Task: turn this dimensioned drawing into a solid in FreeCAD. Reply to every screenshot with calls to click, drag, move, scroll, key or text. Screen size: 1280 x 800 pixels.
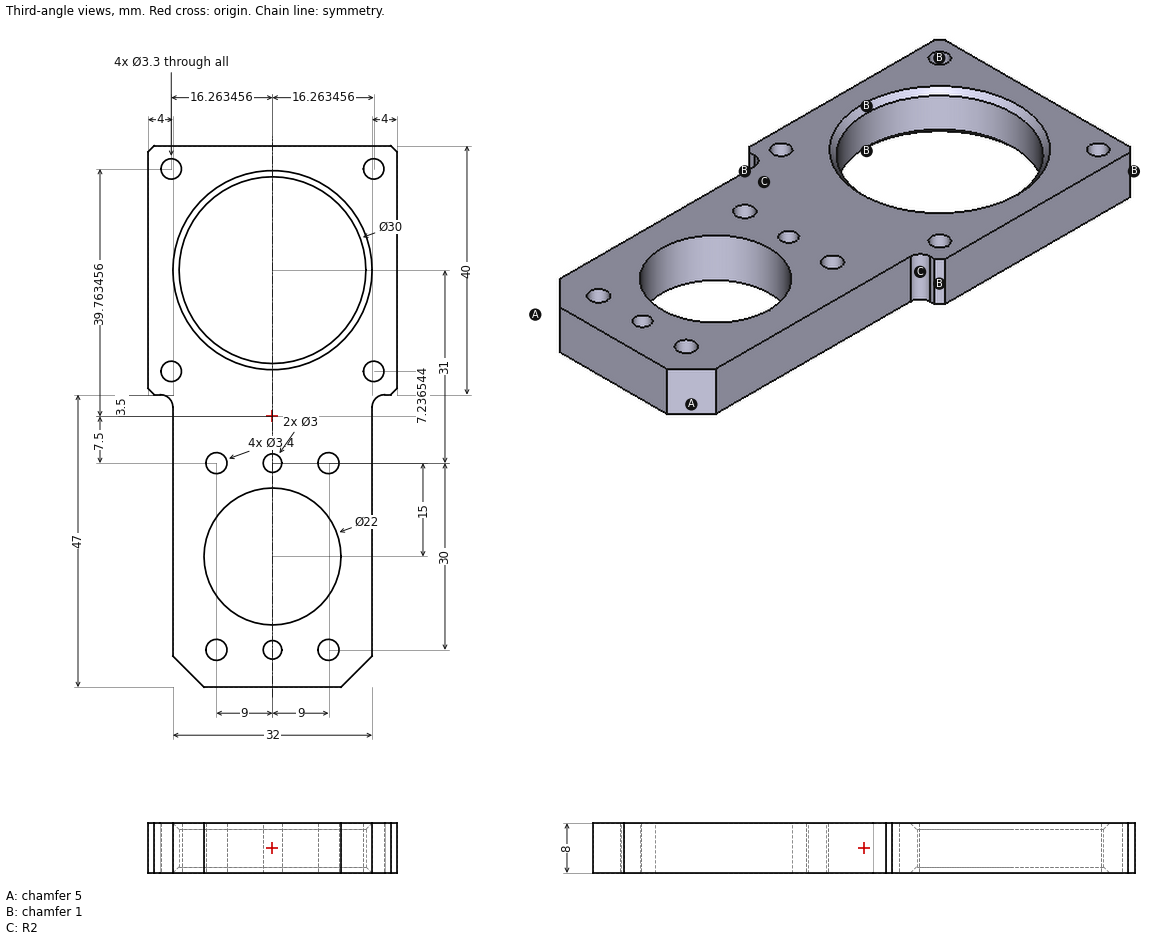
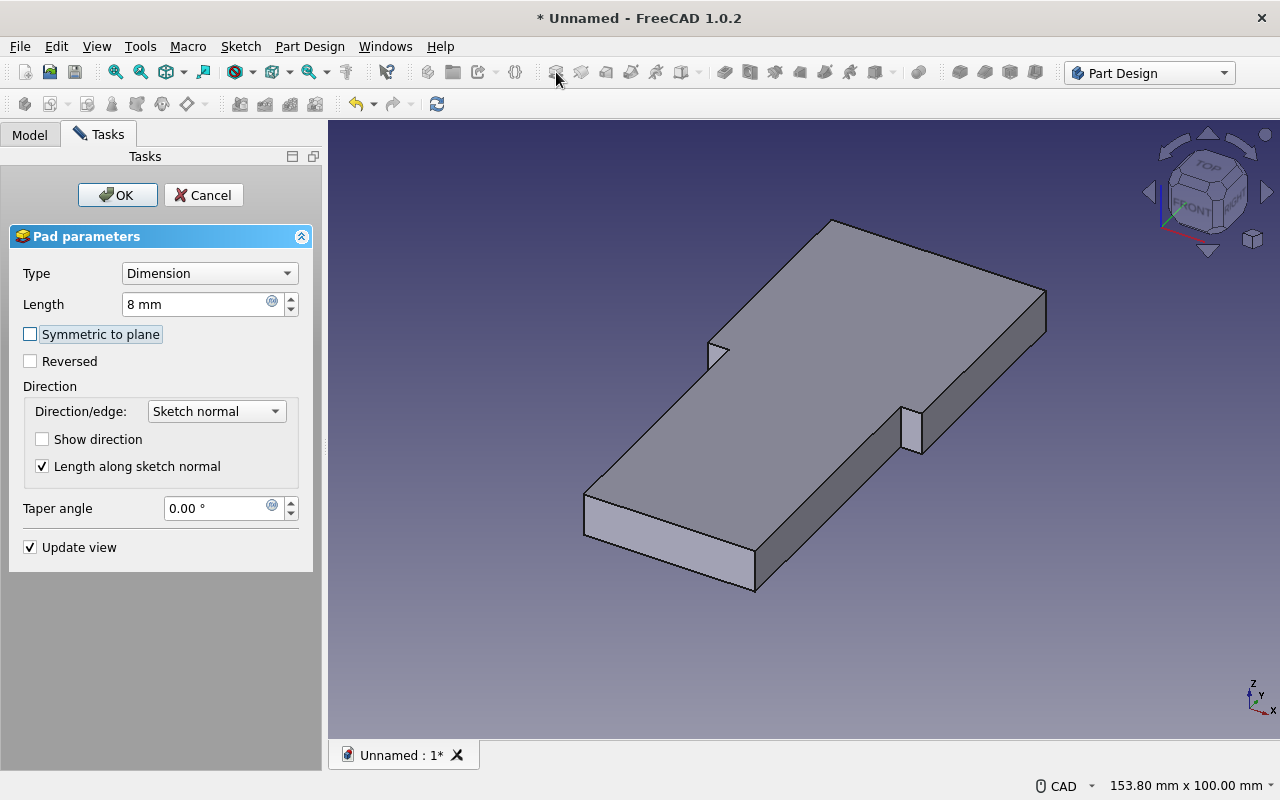
click(31, 334)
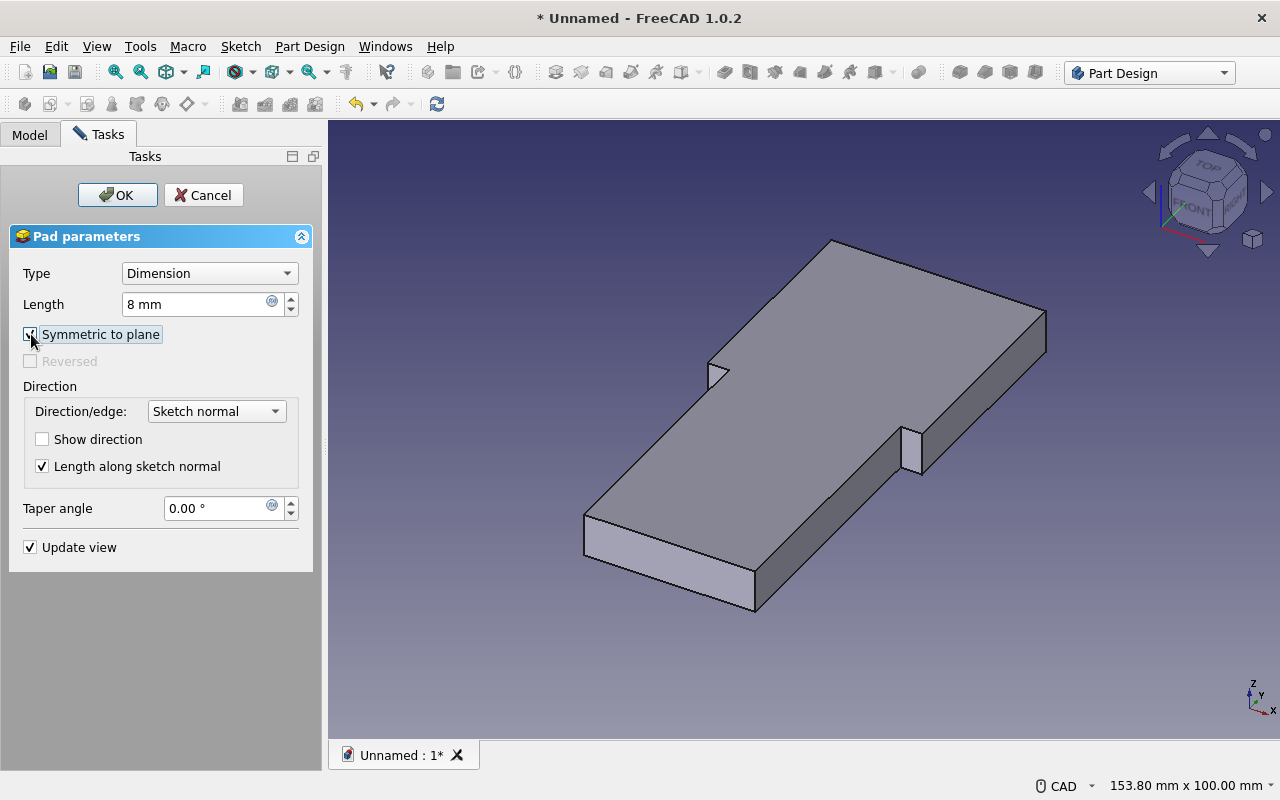
click(118, 195)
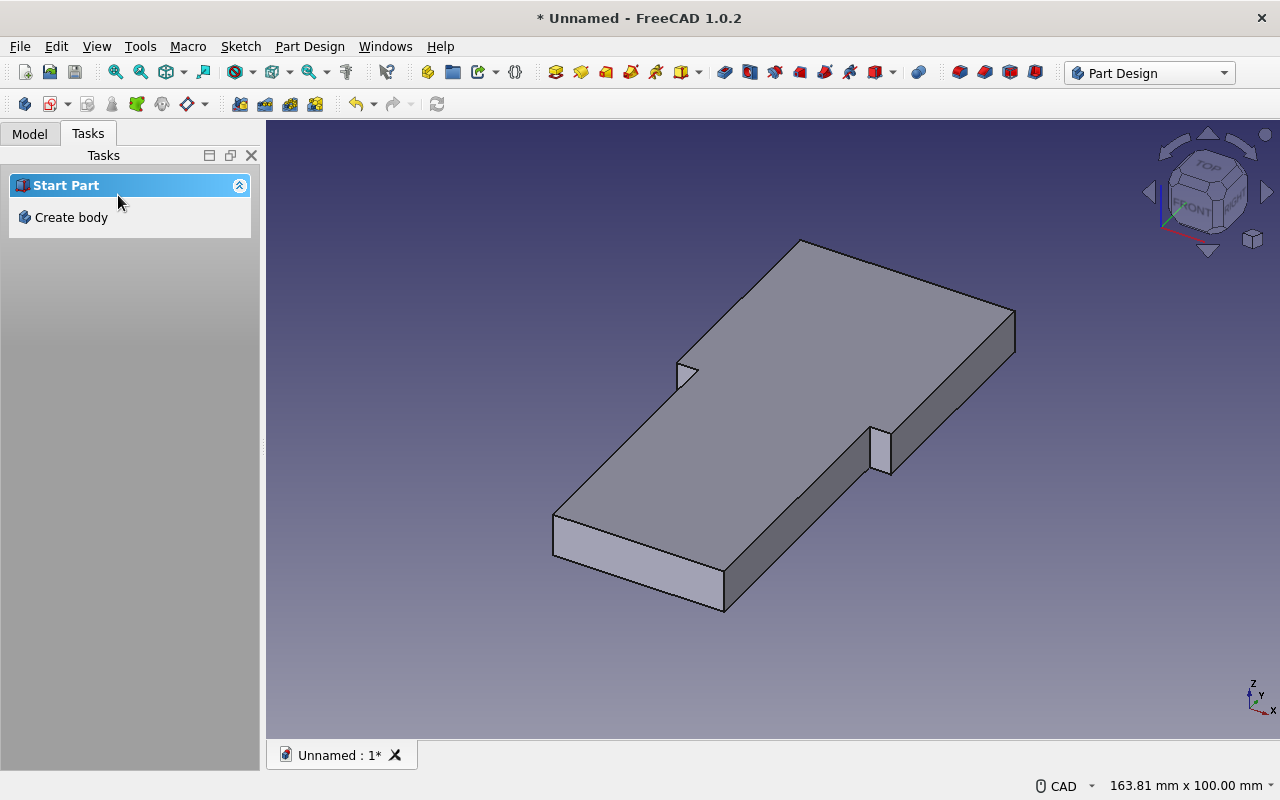
click(850, 332)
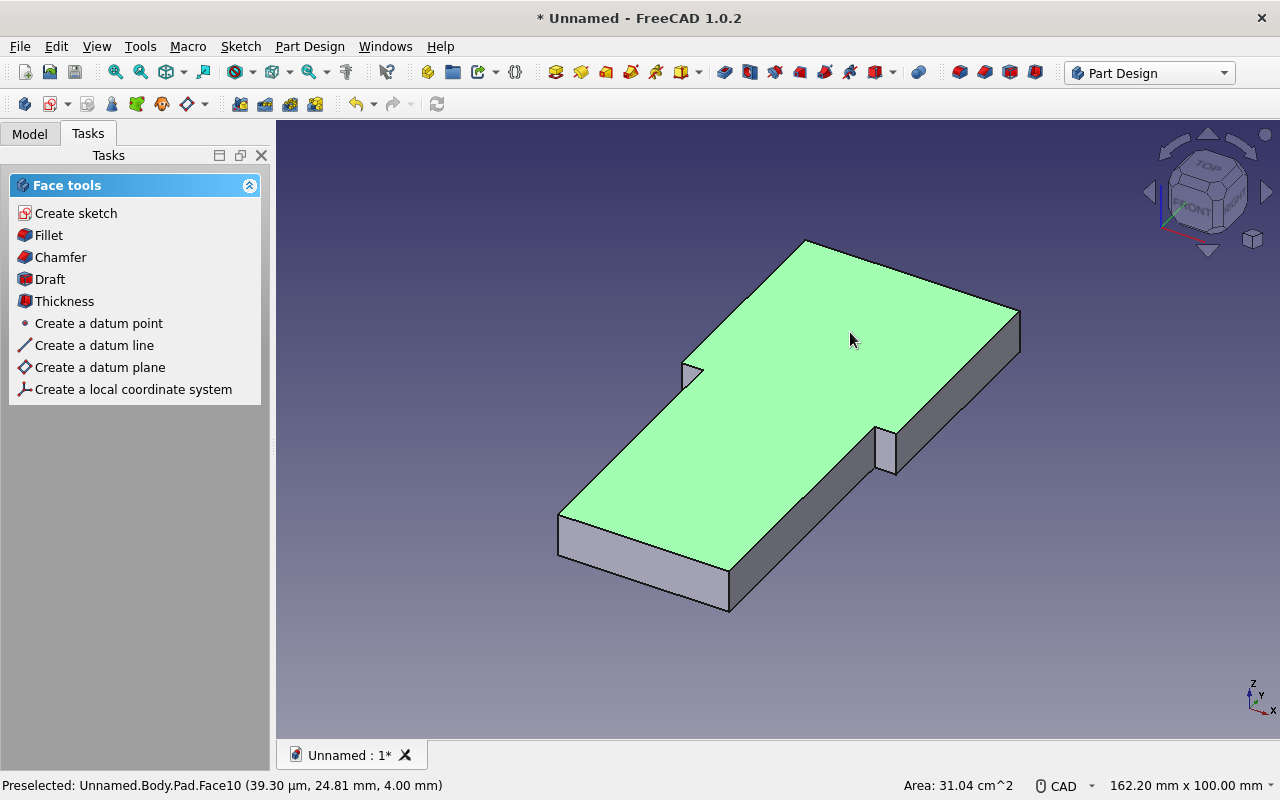
click(50, 104)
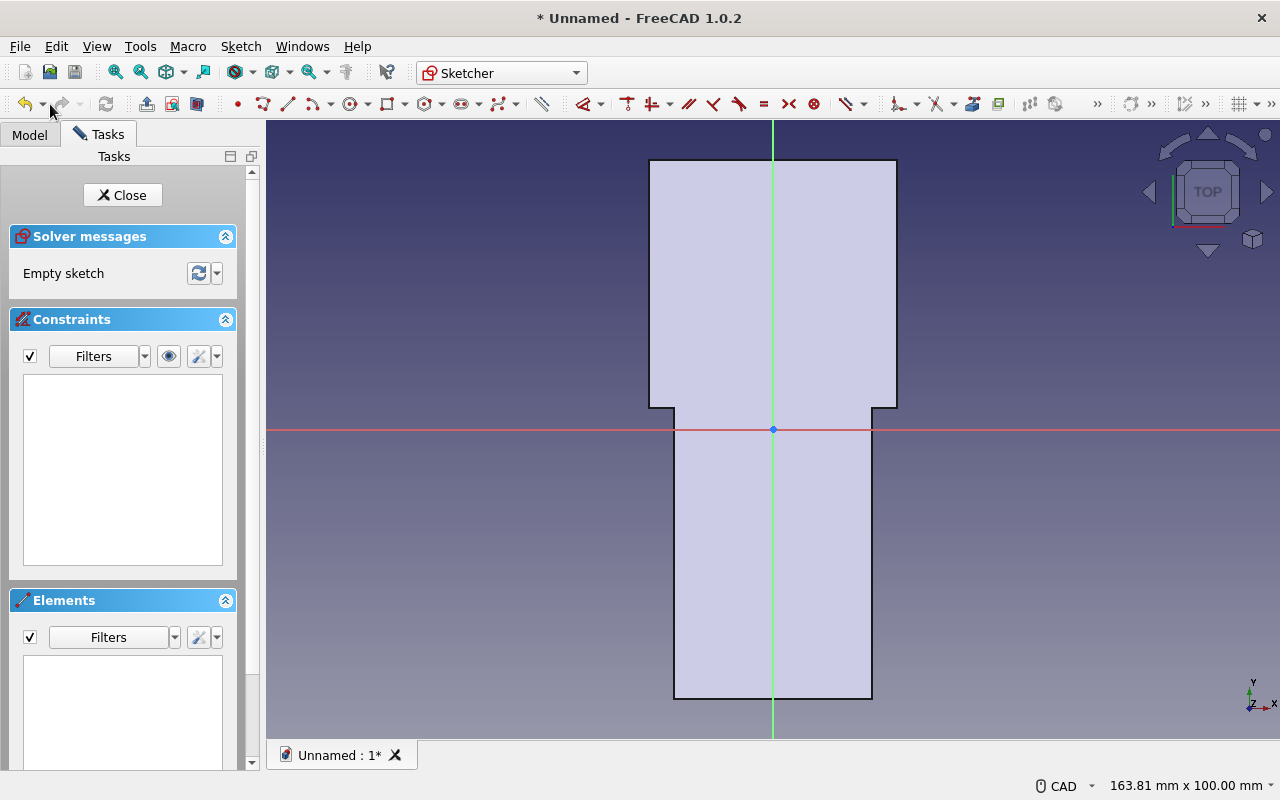
scroll(912, 148, up, 2)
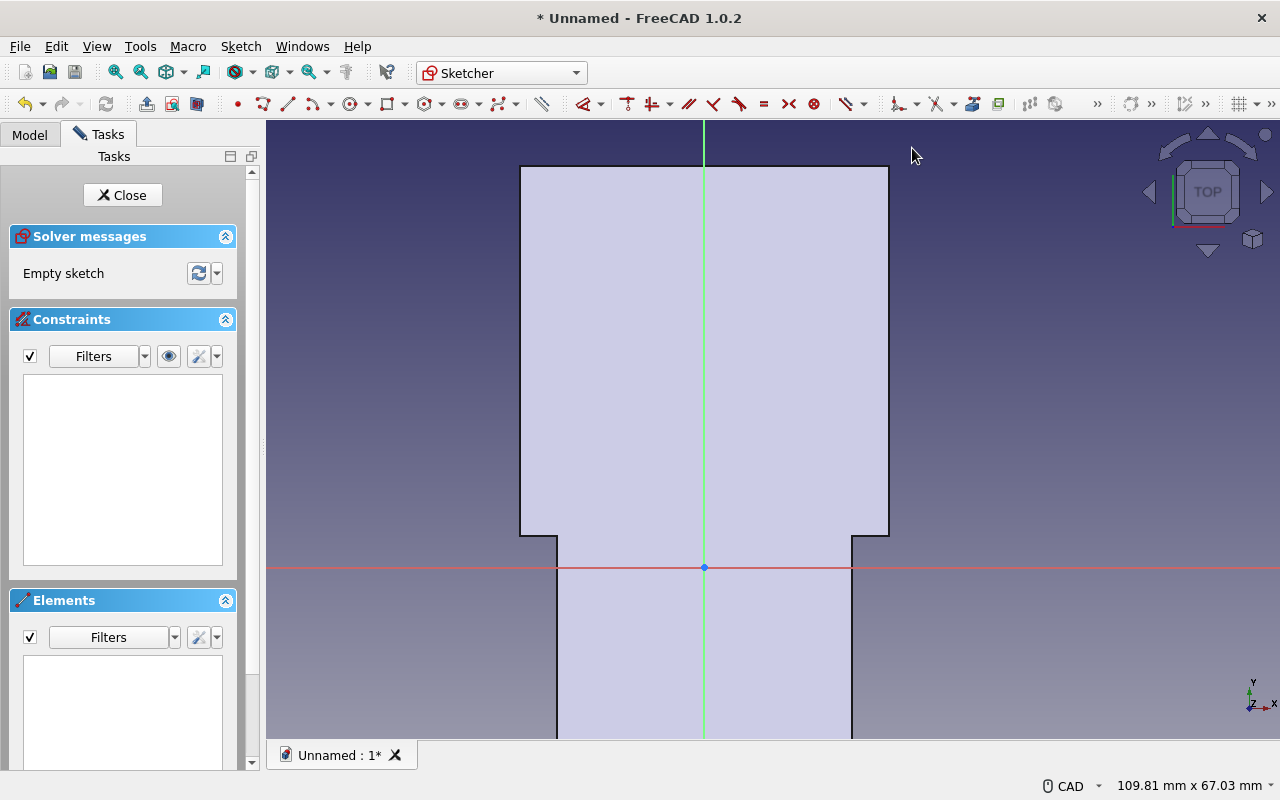
click(350, 104)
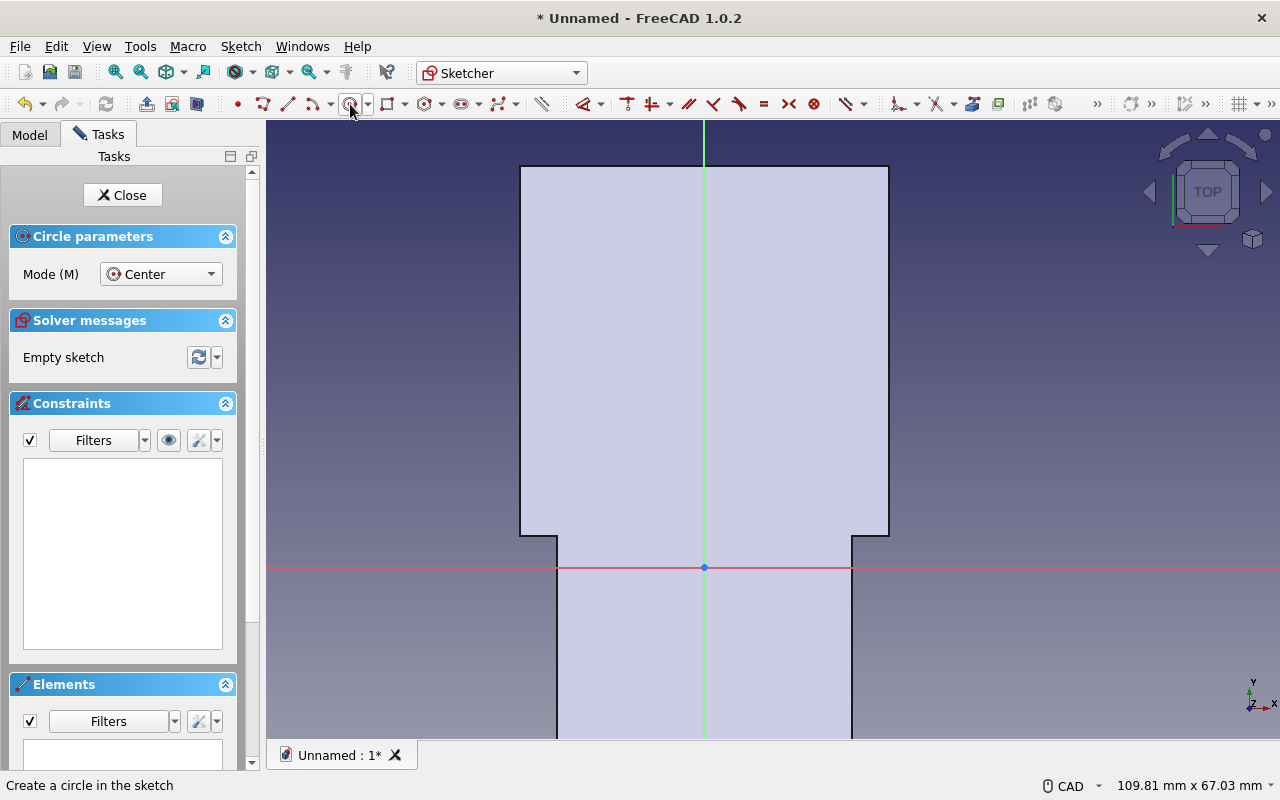
scroll(554, 201, up, 2)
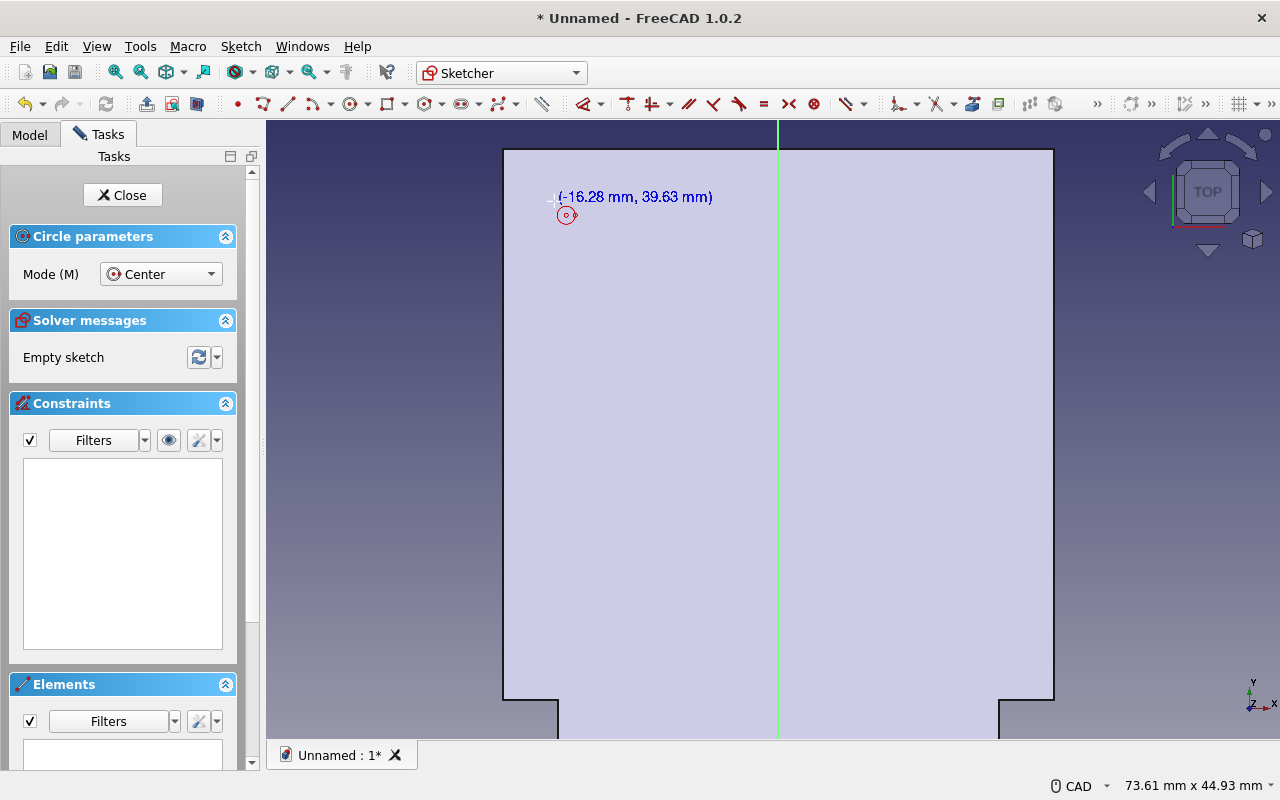
click(554, 201)
click(570, 184)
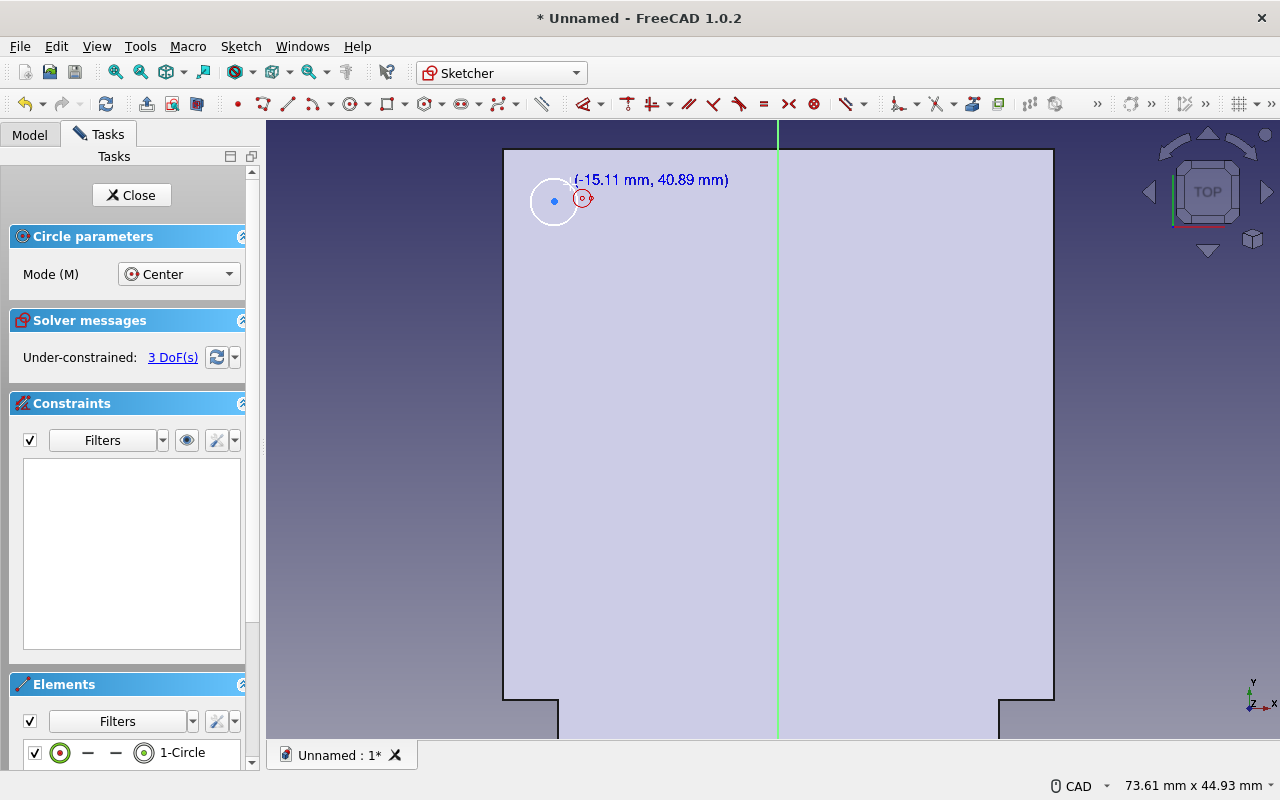
click(1002, 201)
click(1018, 184)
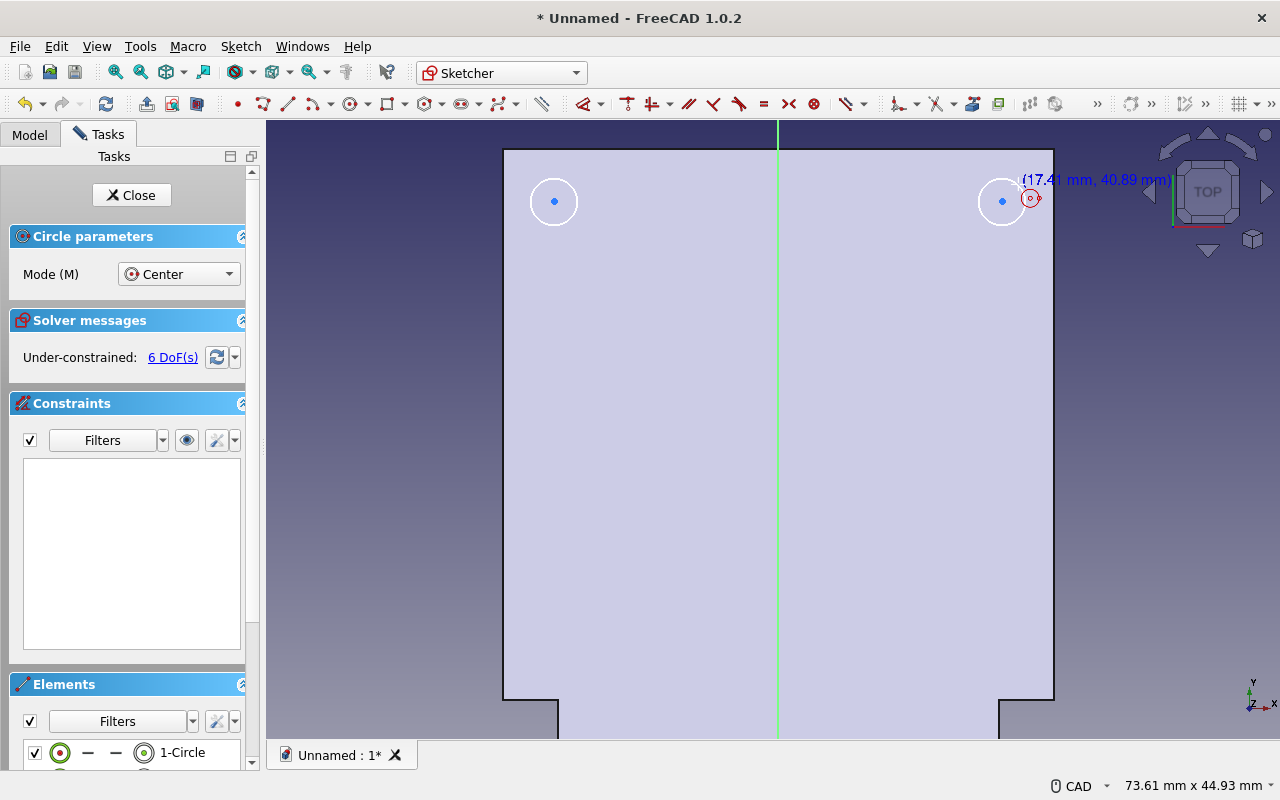
click(1002, 649)
click(1018, 633)